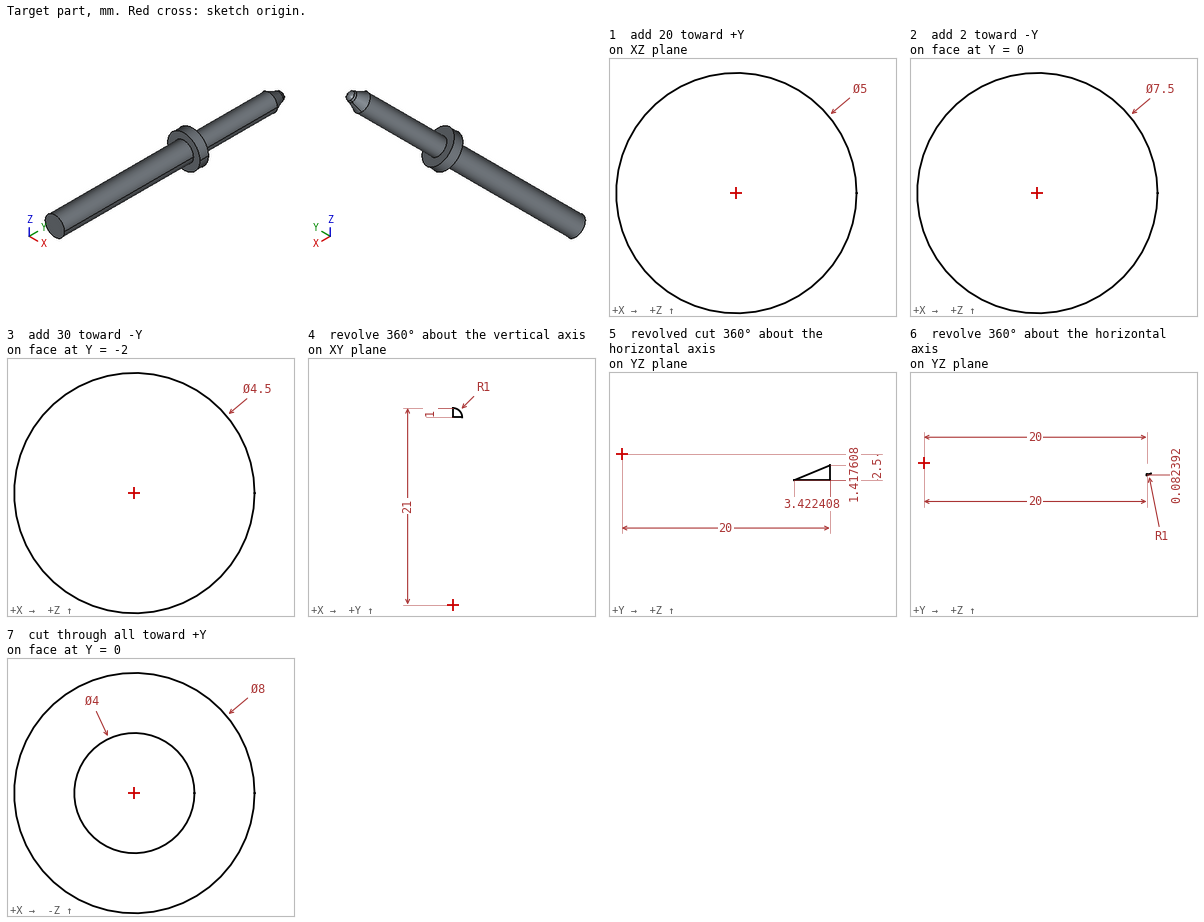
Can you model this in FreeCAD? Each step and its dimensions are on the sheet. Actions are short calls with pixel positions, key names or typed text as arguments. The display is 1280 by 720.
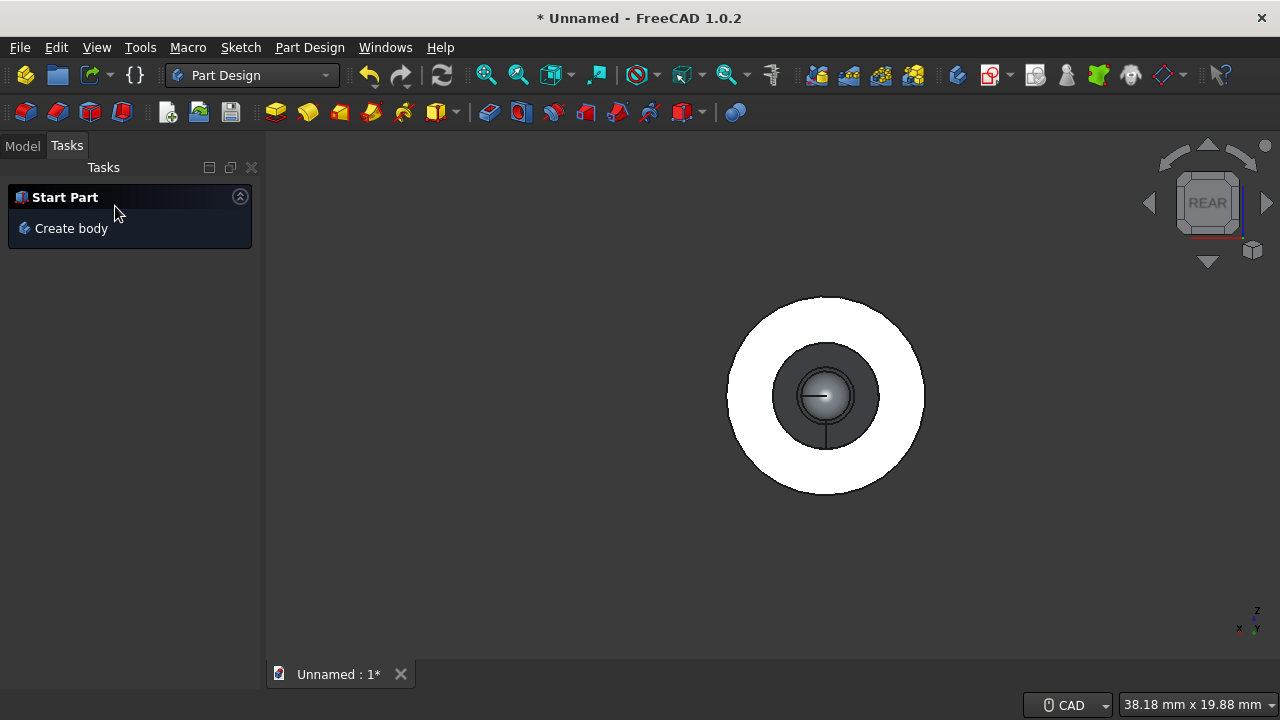
key(0)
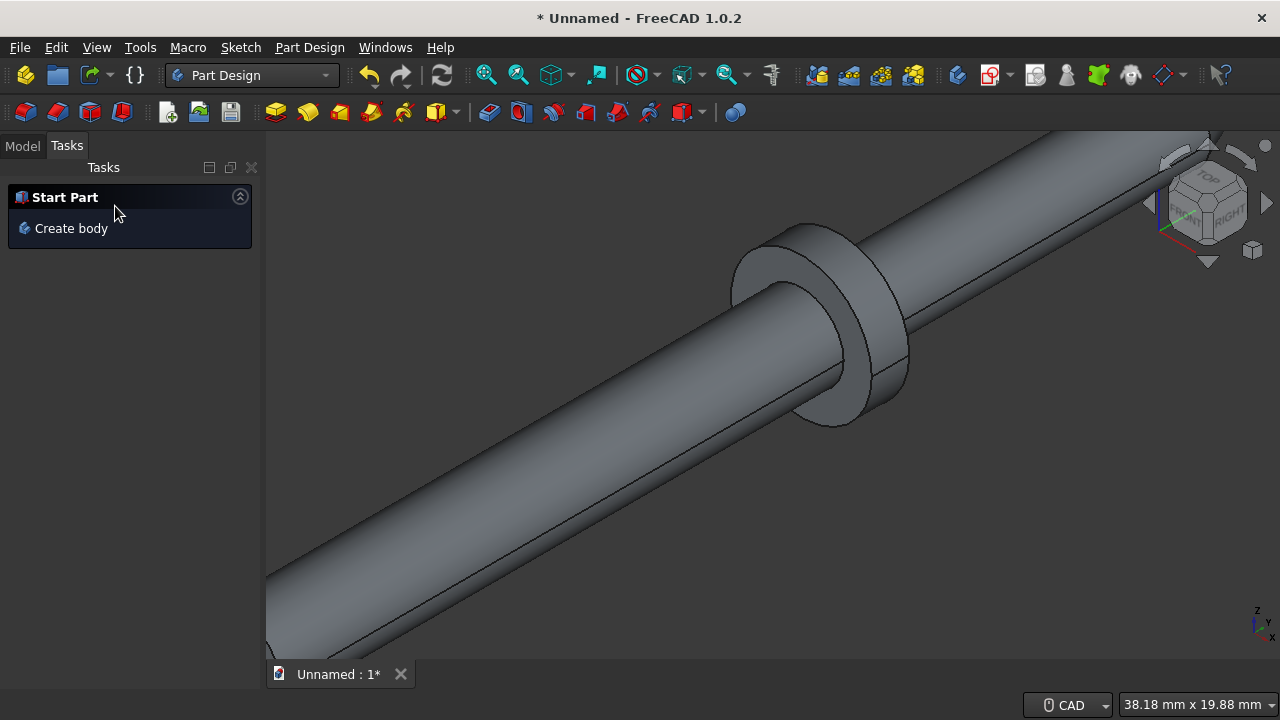
click(488, 76)